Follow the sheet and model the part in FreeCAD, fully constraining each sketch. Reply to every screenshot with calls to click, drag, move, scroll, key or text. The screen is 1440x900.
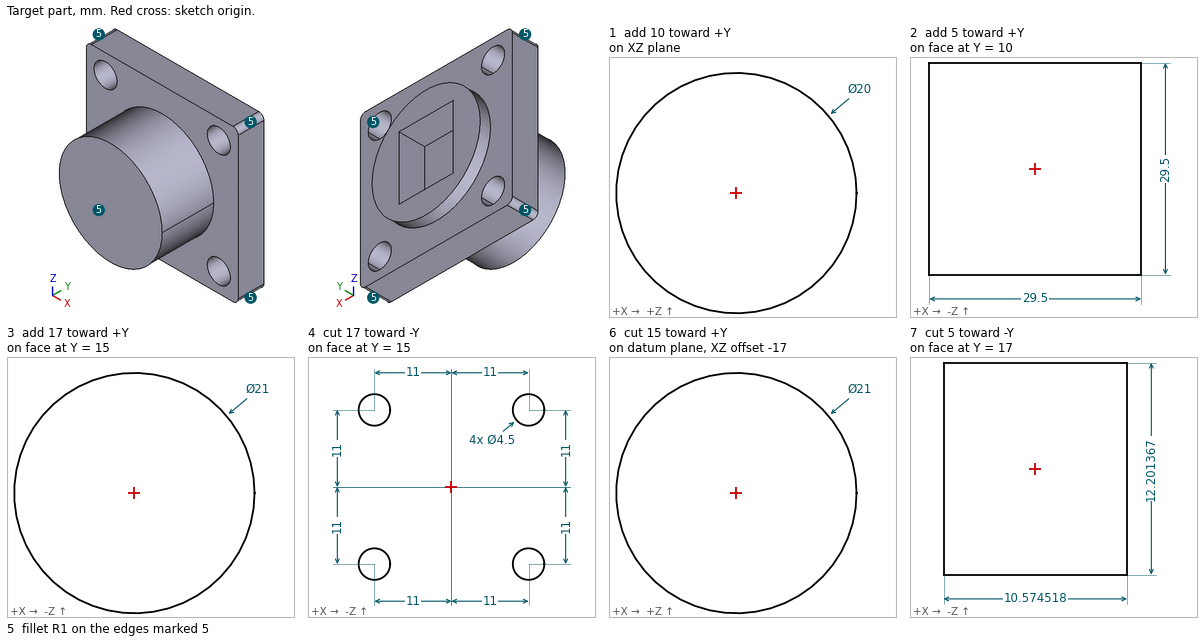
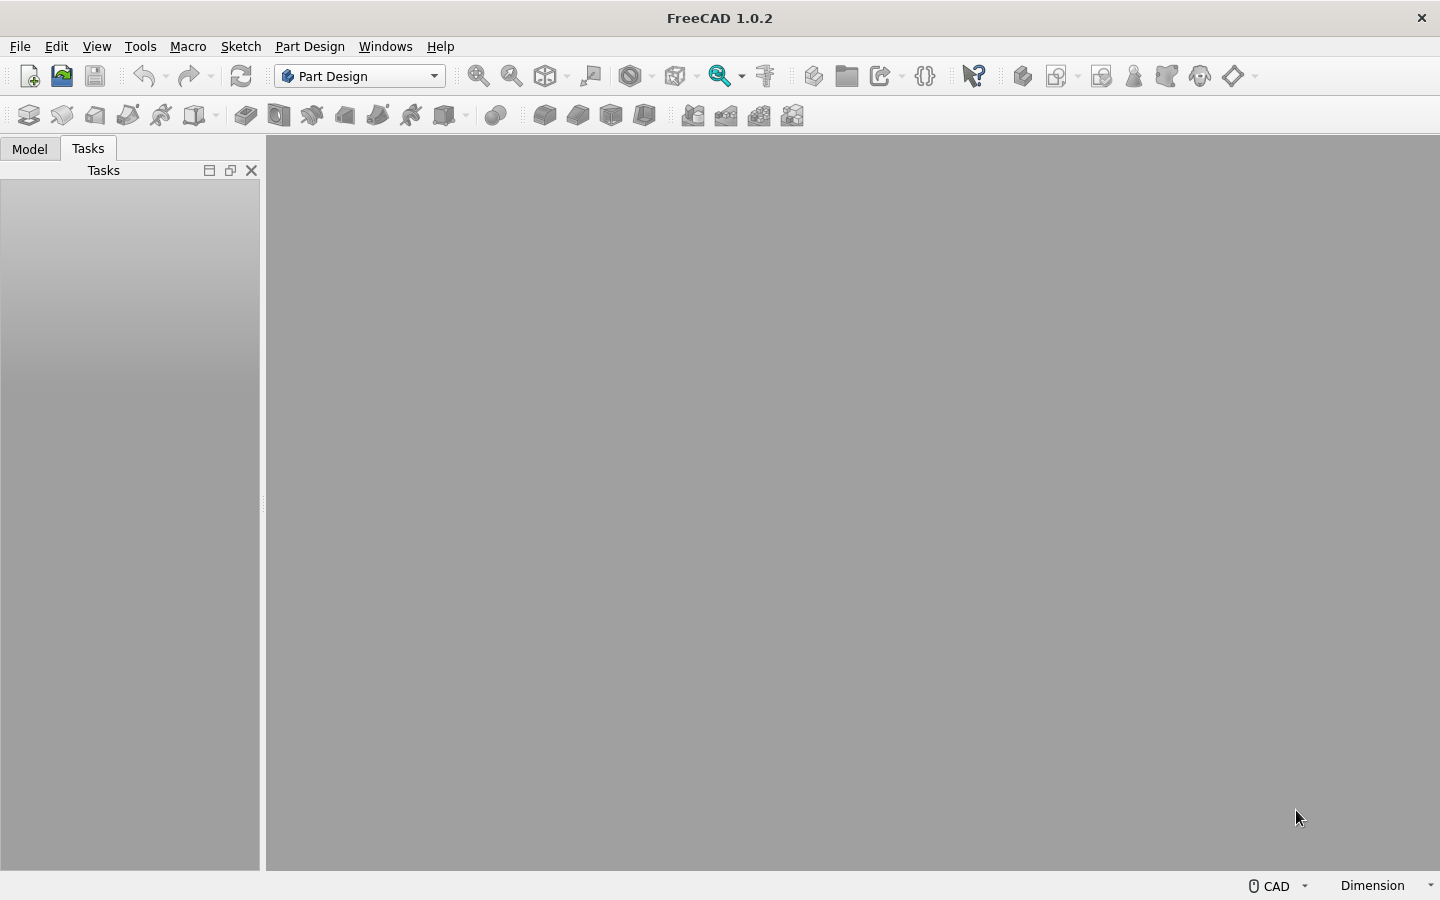
key(ctrl+n)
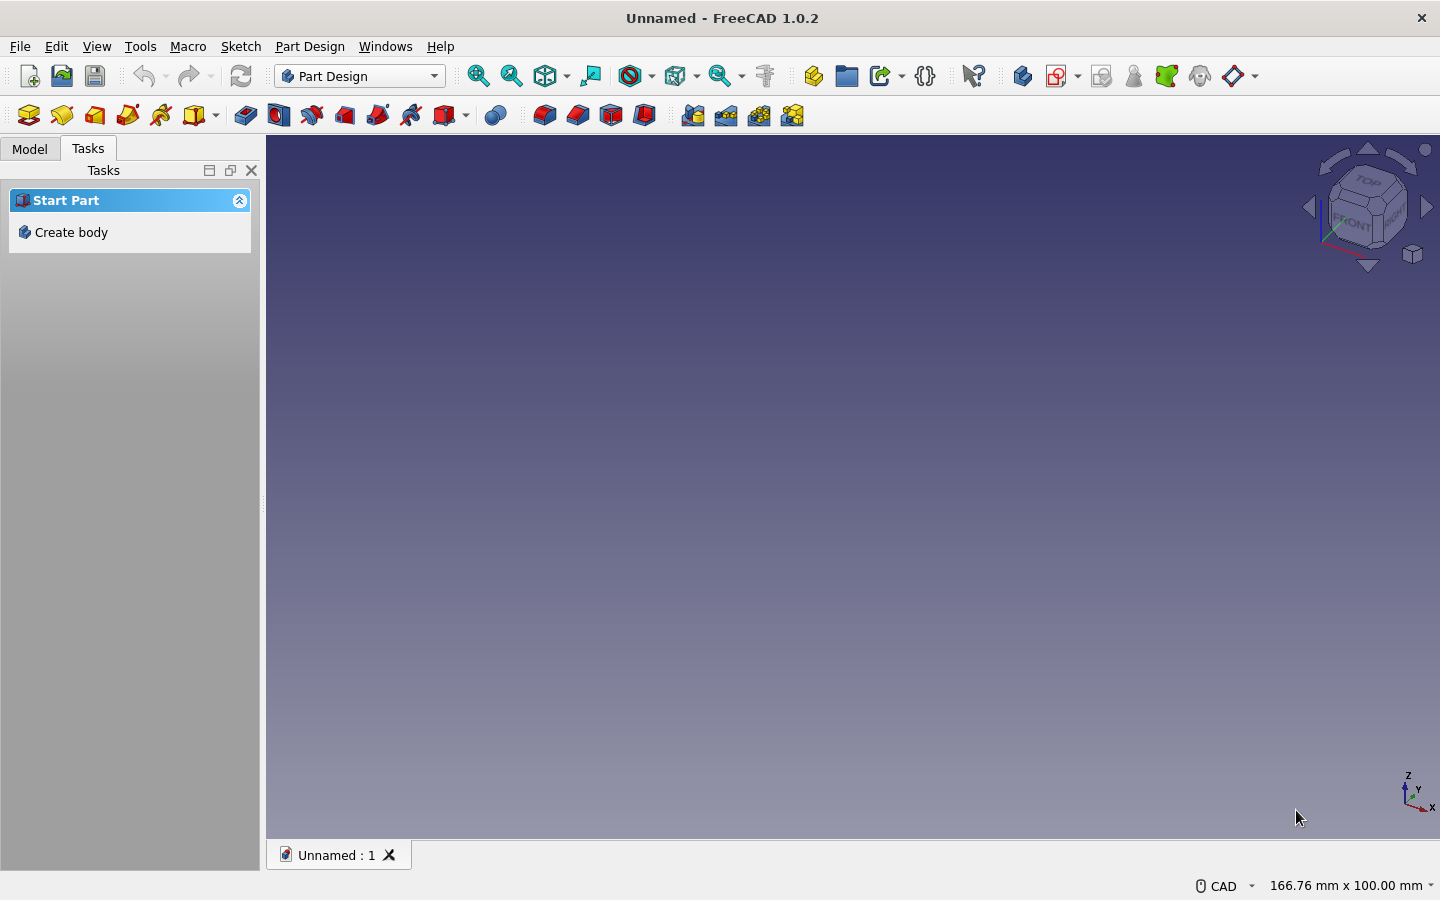
click(1056, 76)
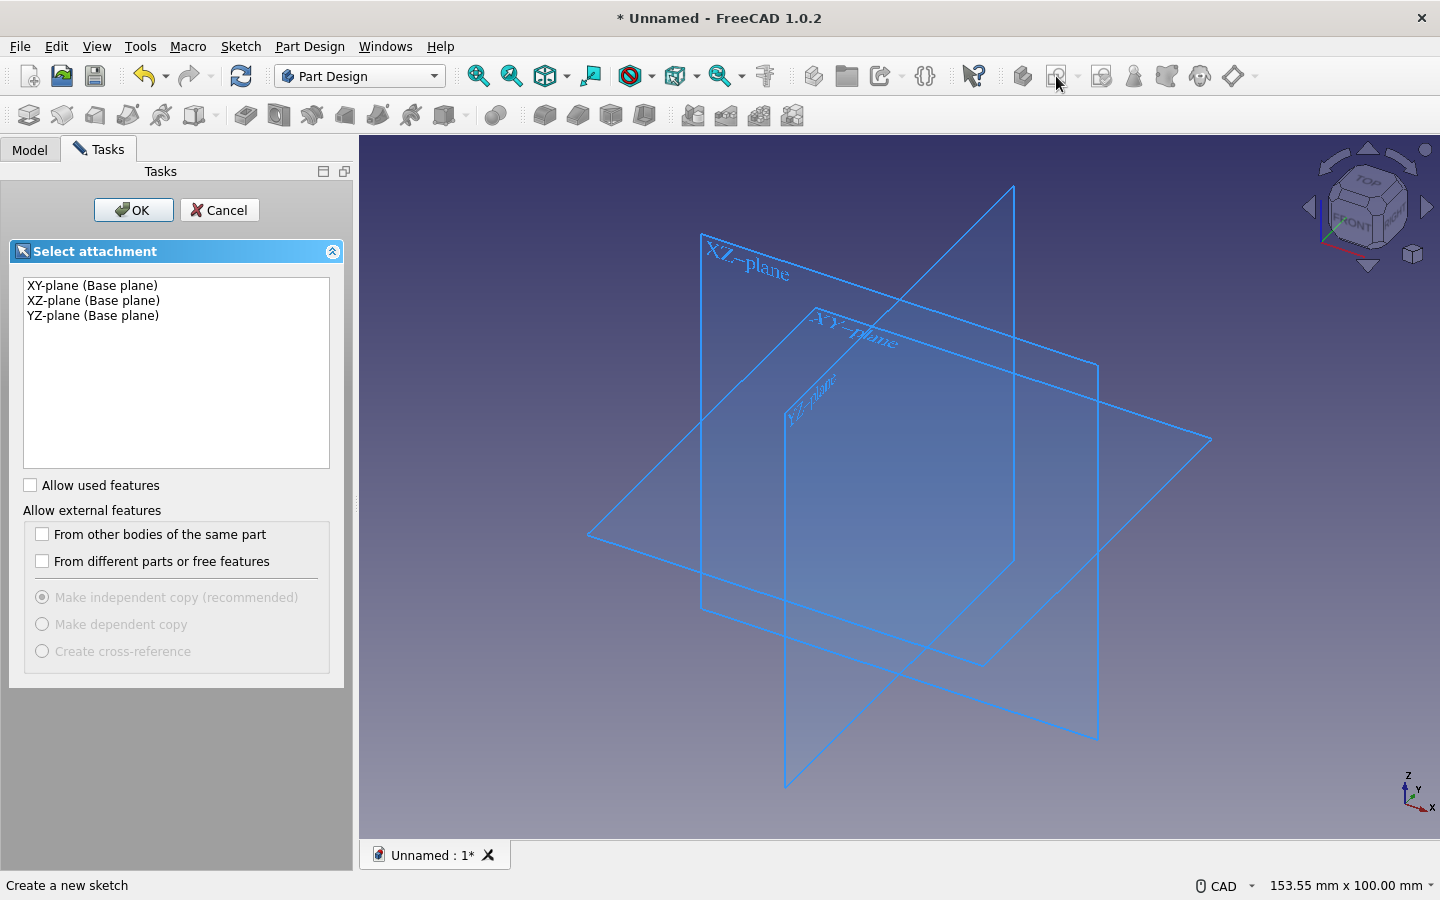
click(84, 300)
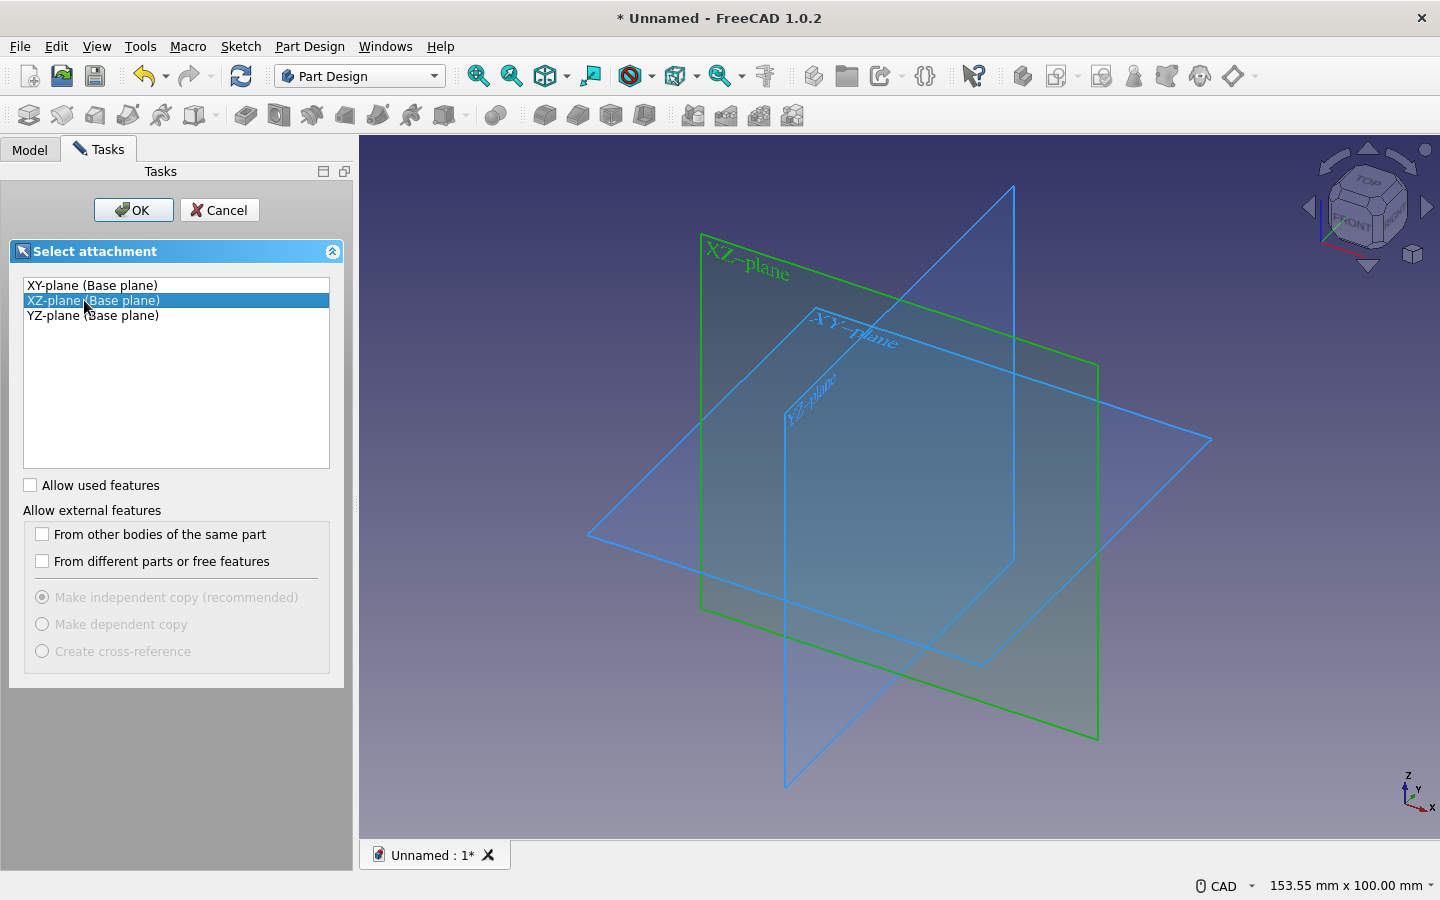
click(134, 210)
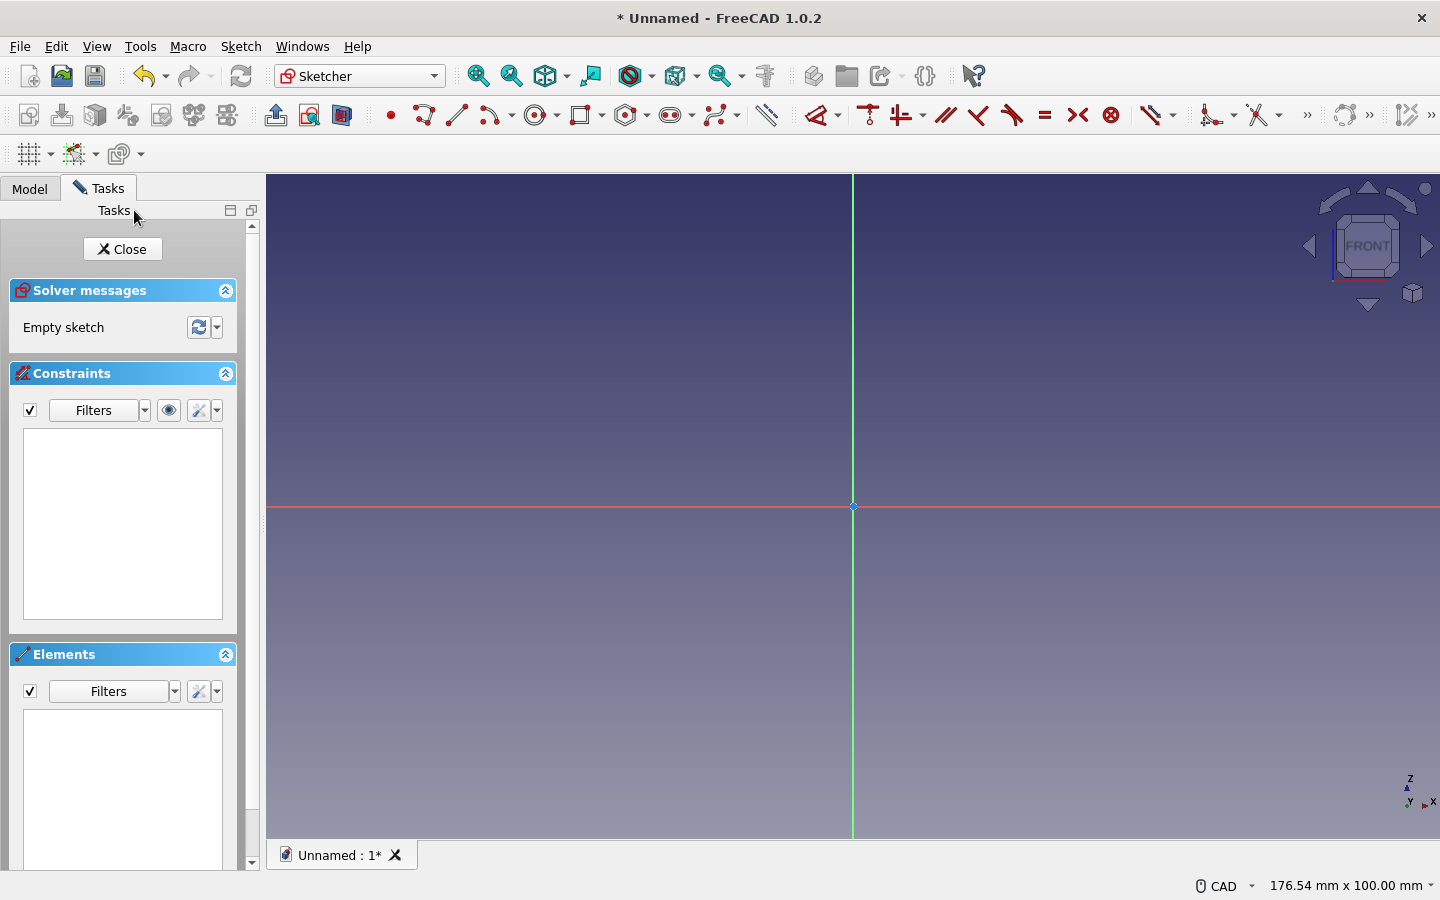
scroll(883, 506, up, 6)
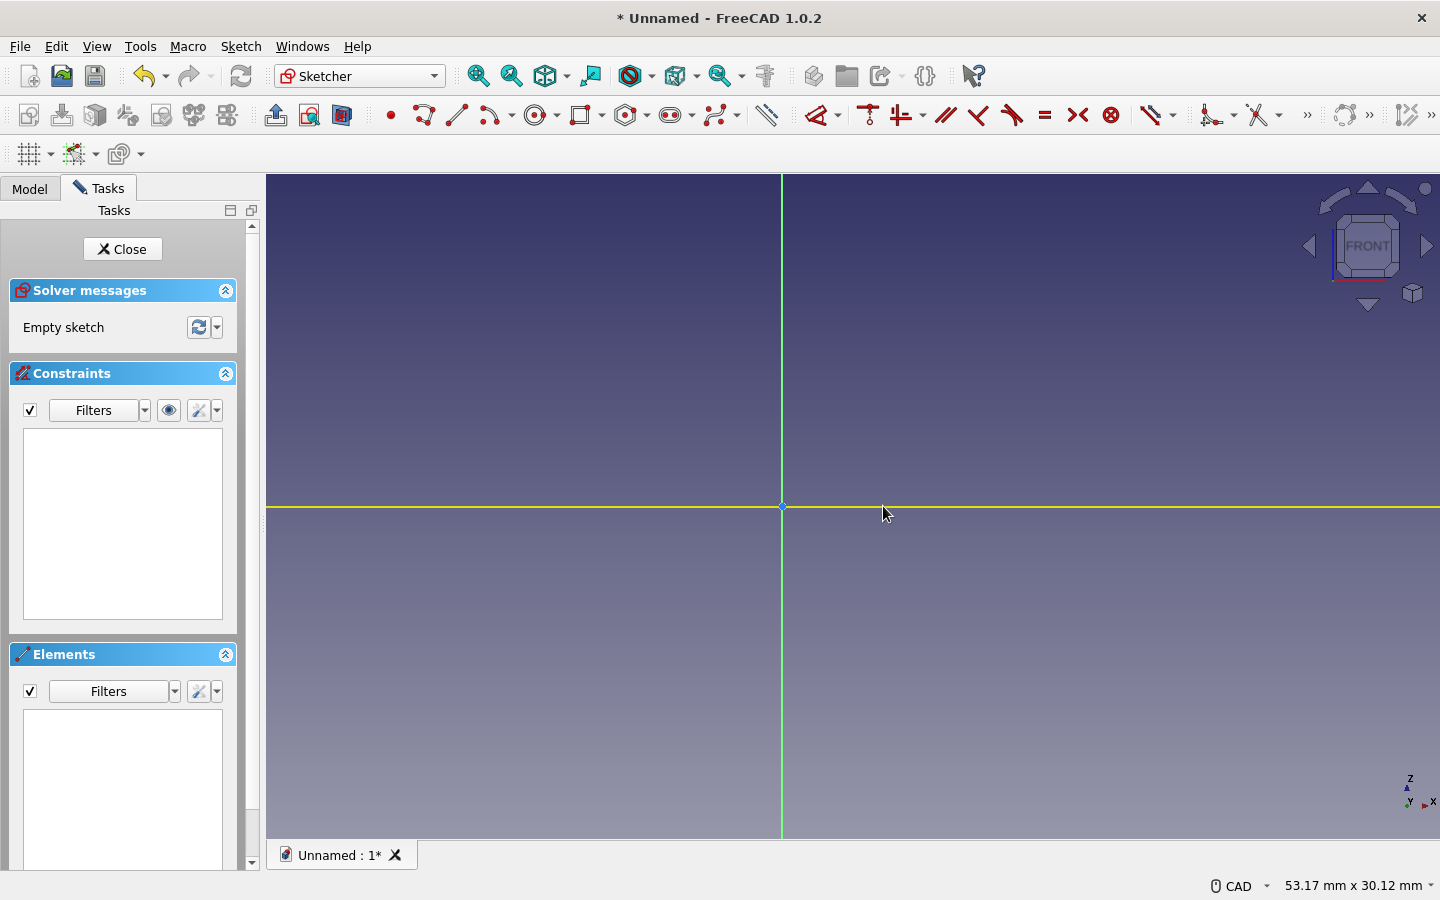
click(534, 116)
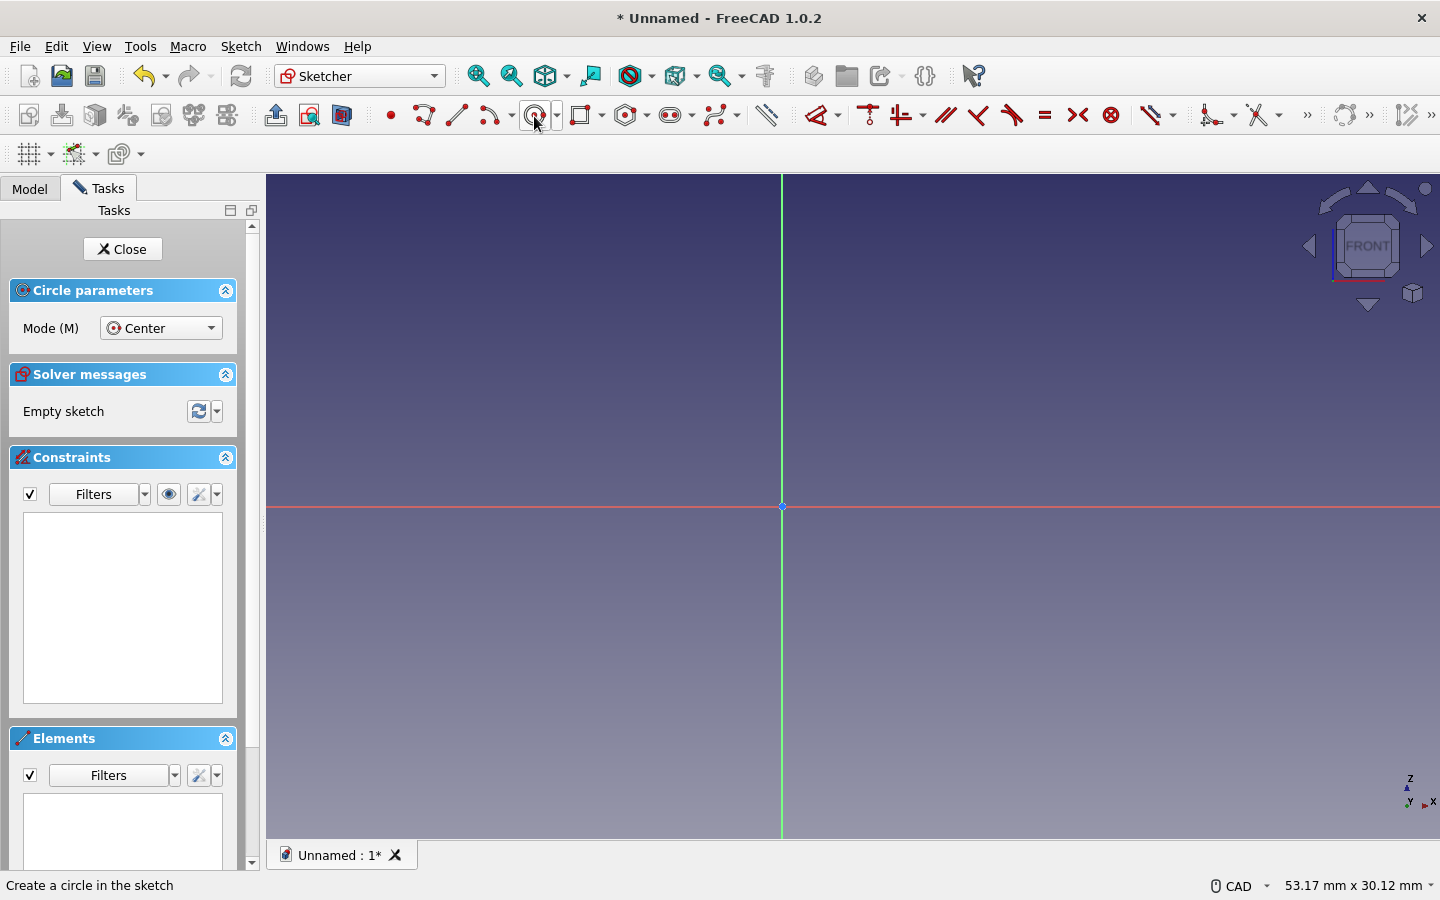
click(782, 506)
click(938, 350)
key(Escape)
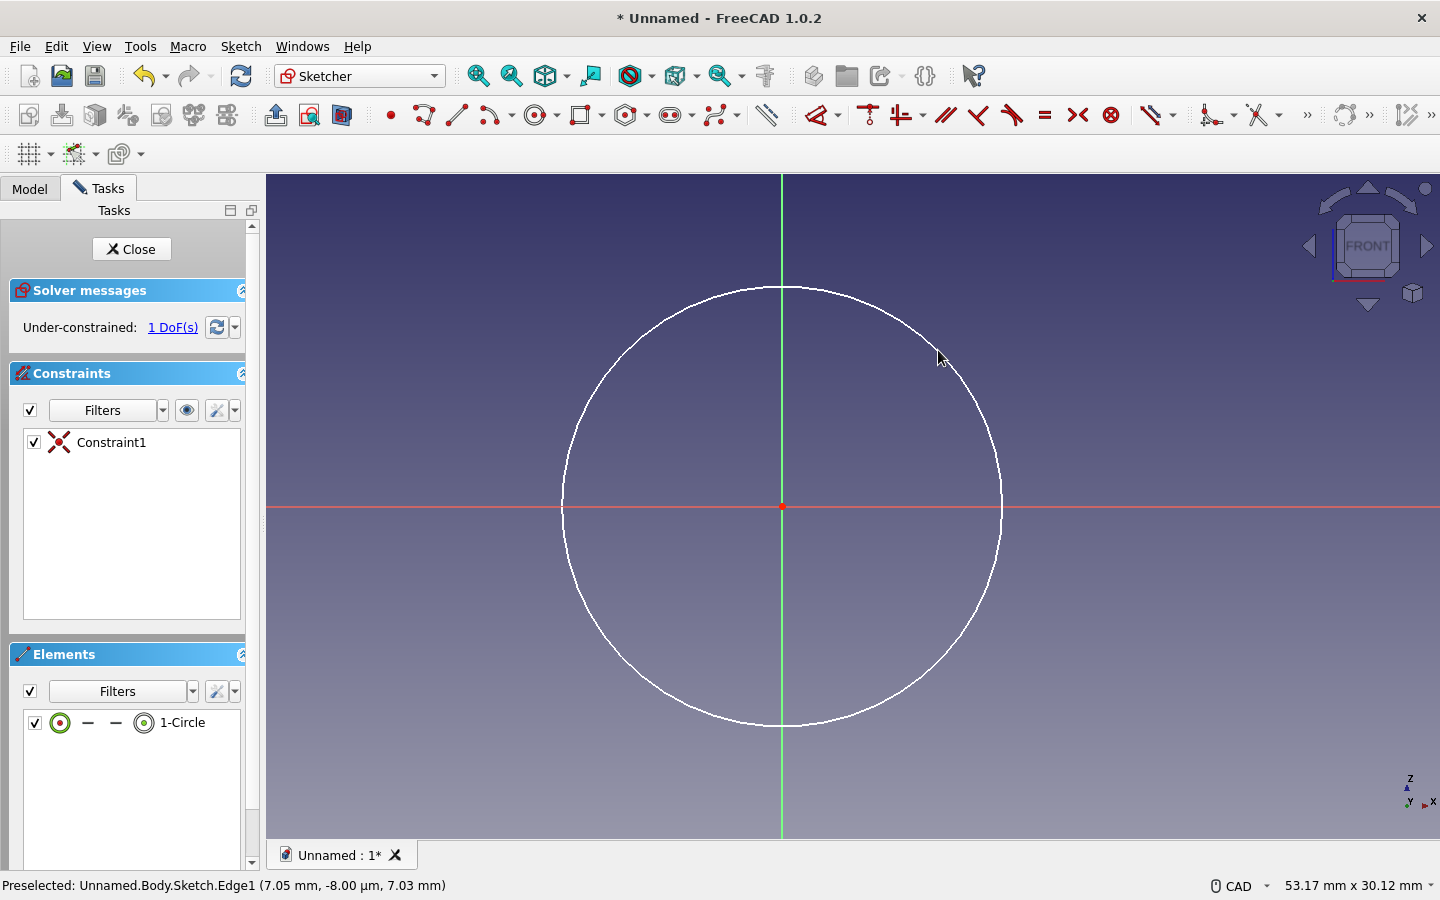
click(937, 350)